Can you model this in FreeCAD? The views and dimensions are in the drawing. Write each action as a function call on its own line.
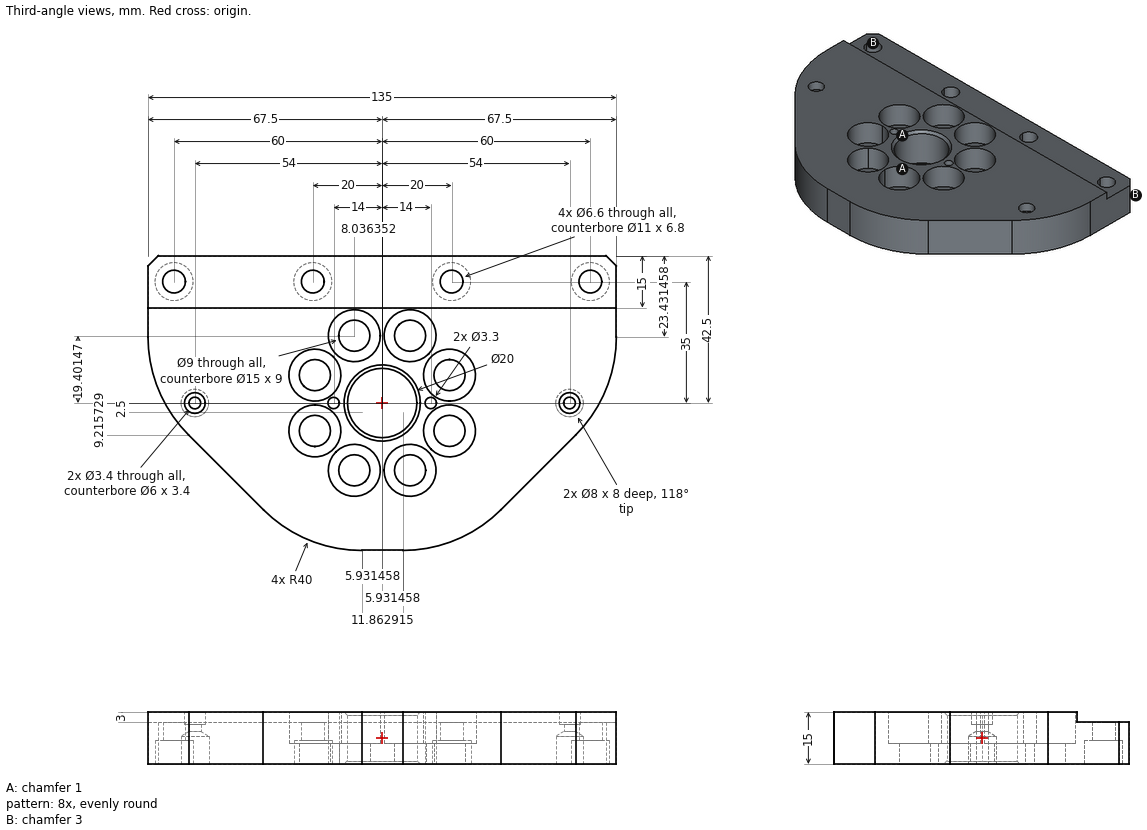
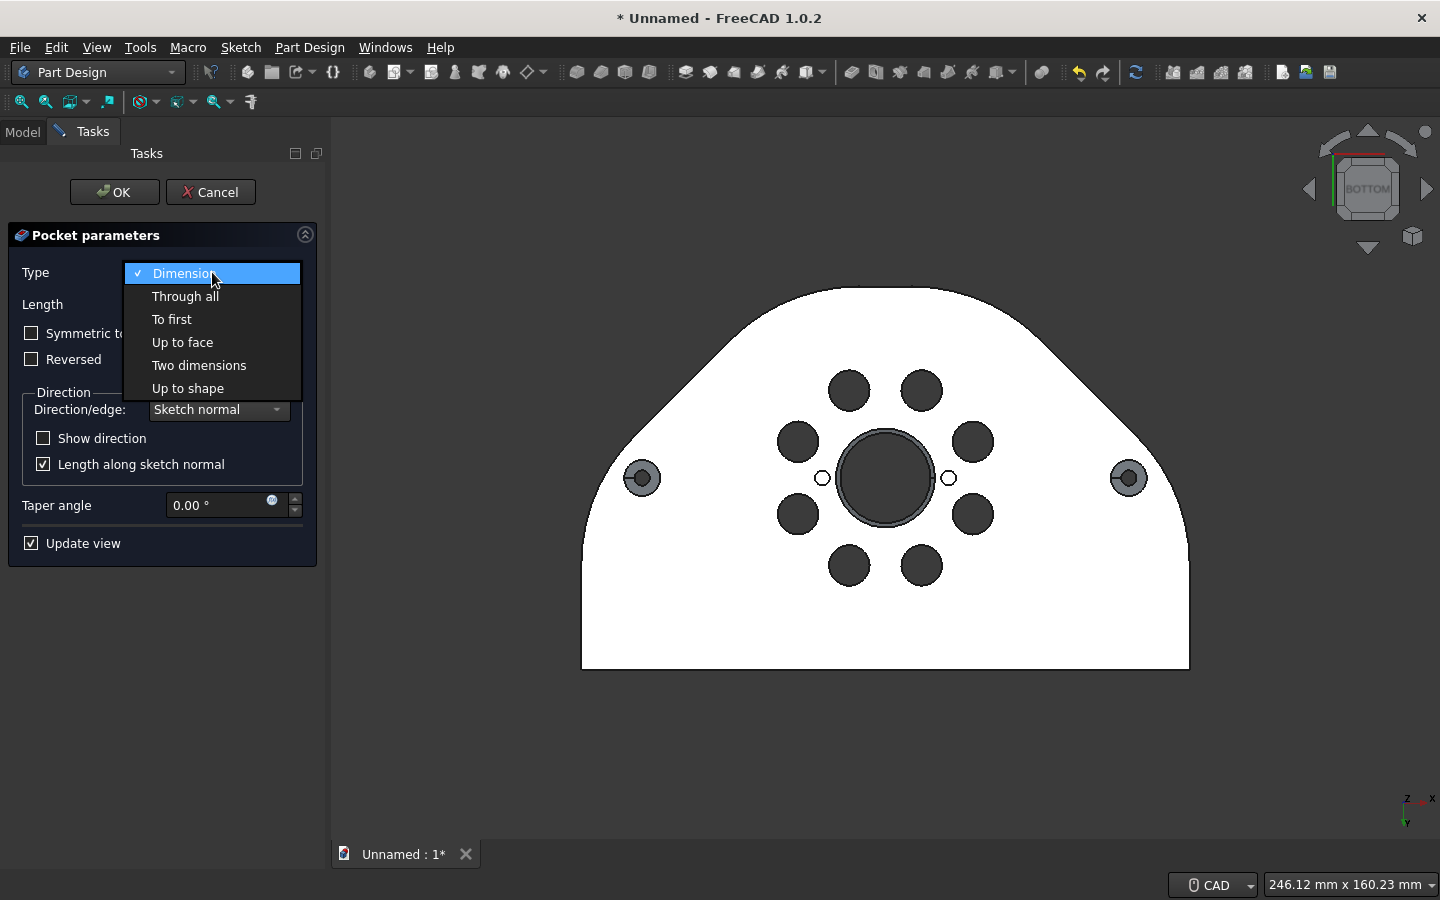
click(212, 296)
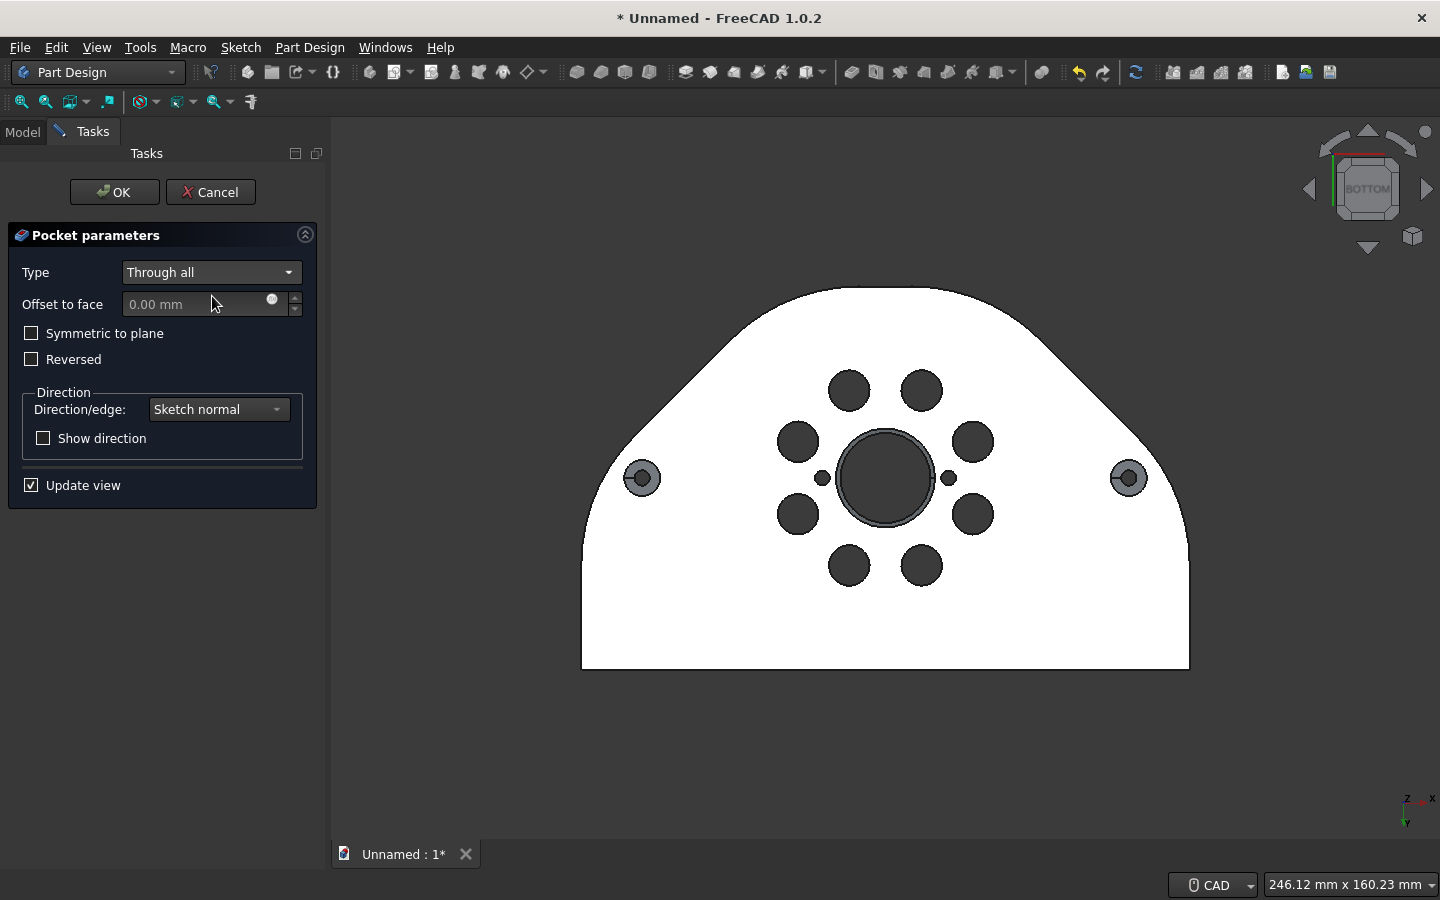
click(115, 192)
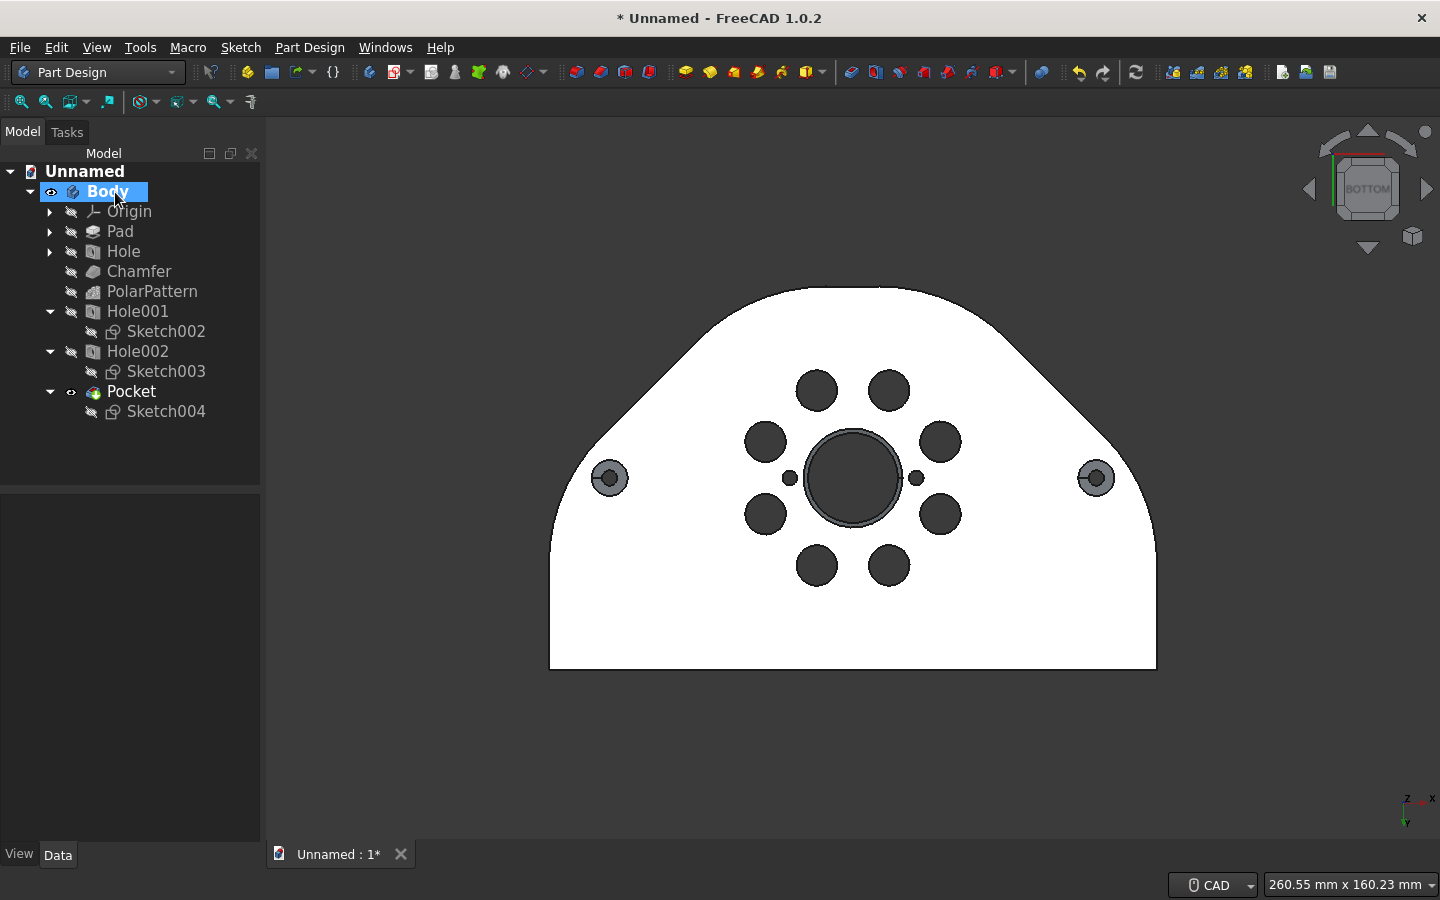
key(0)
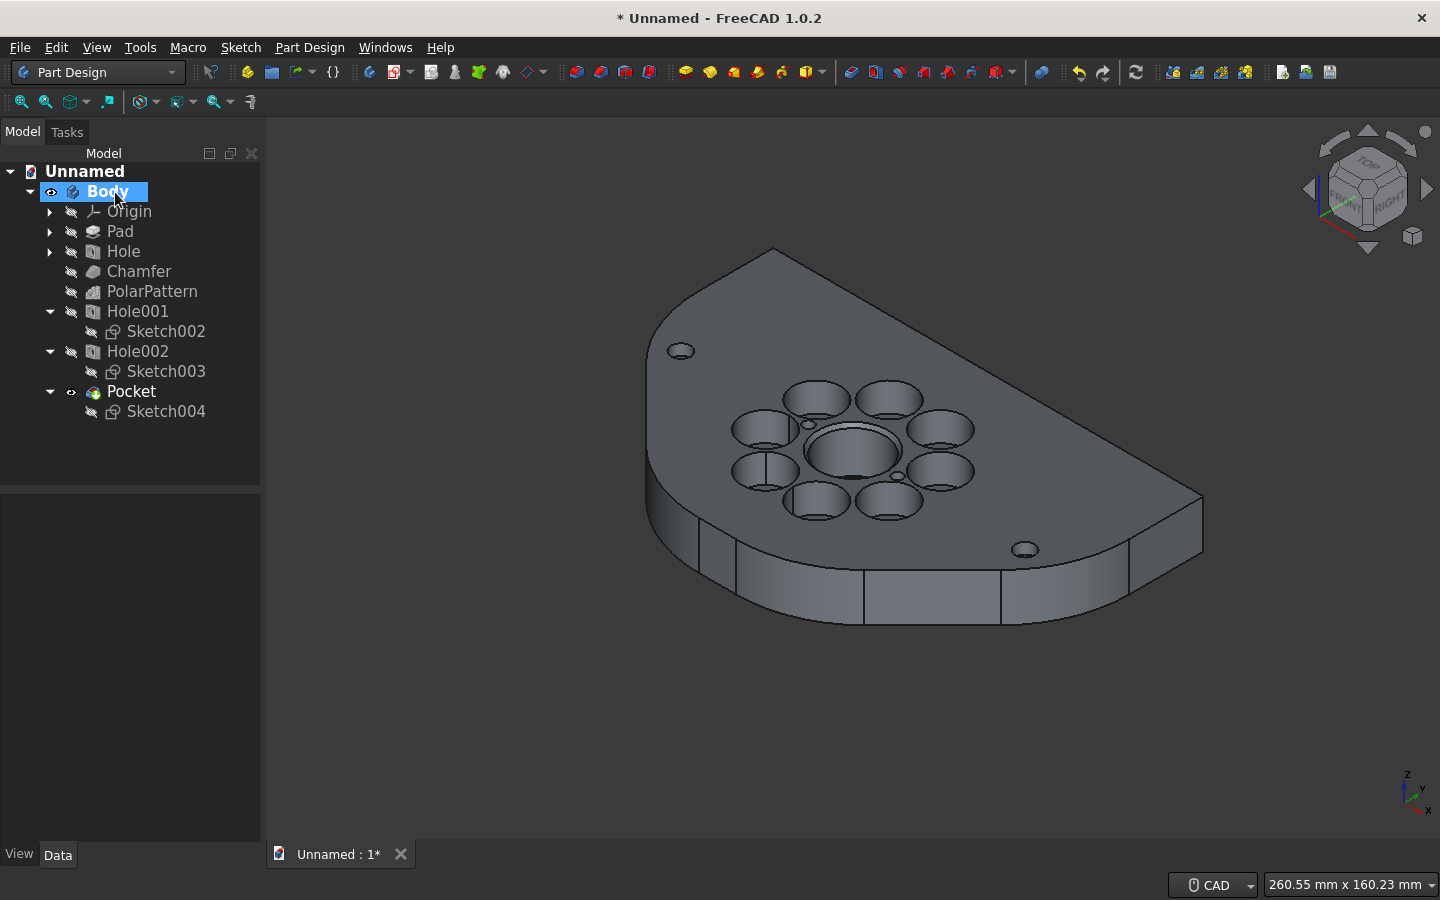
click(1053, 476)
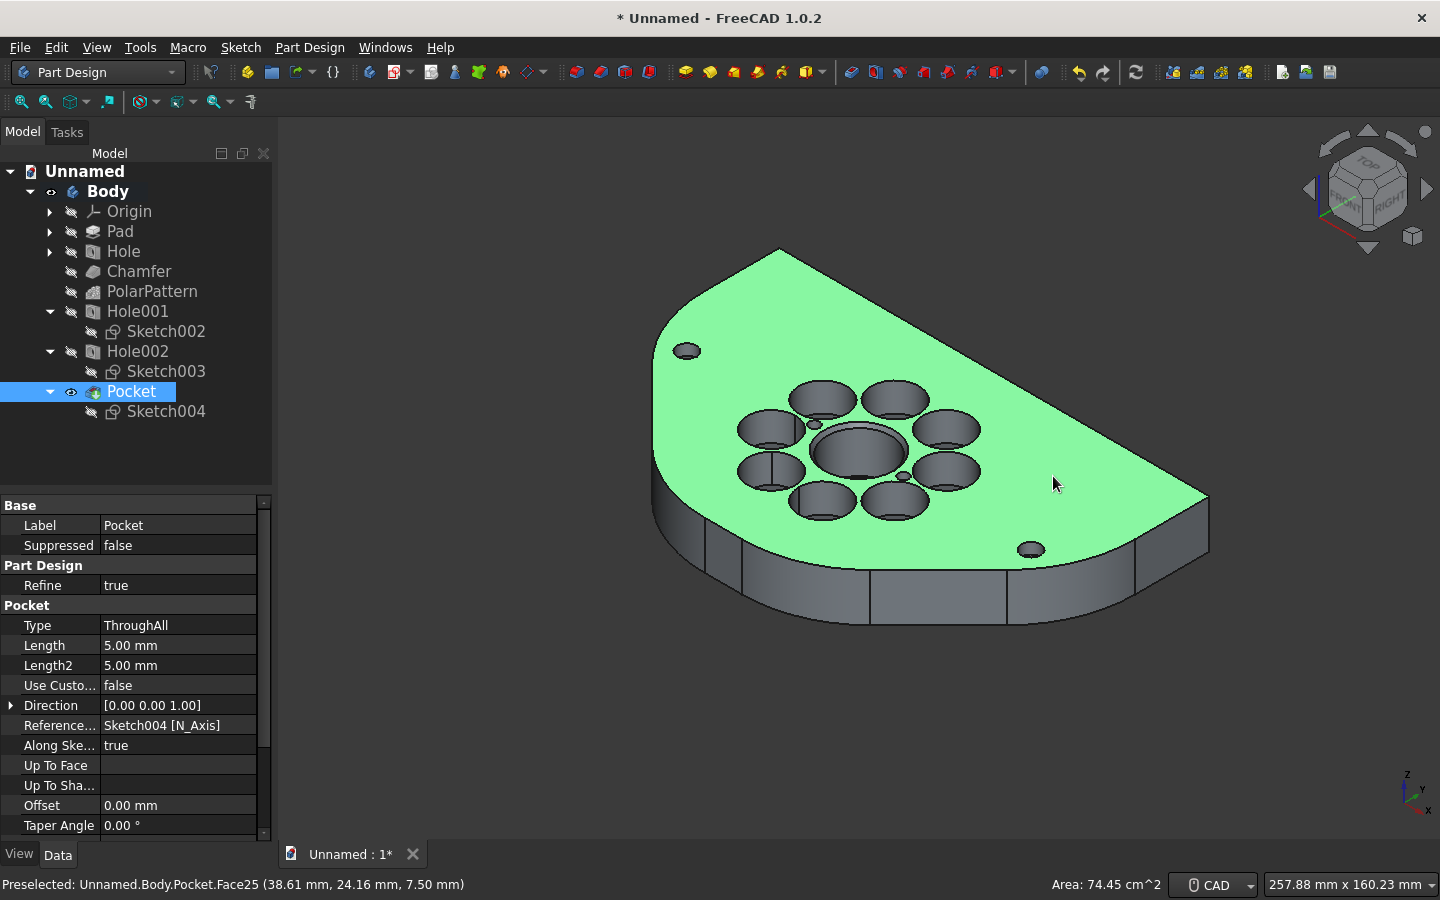
click(394, 72)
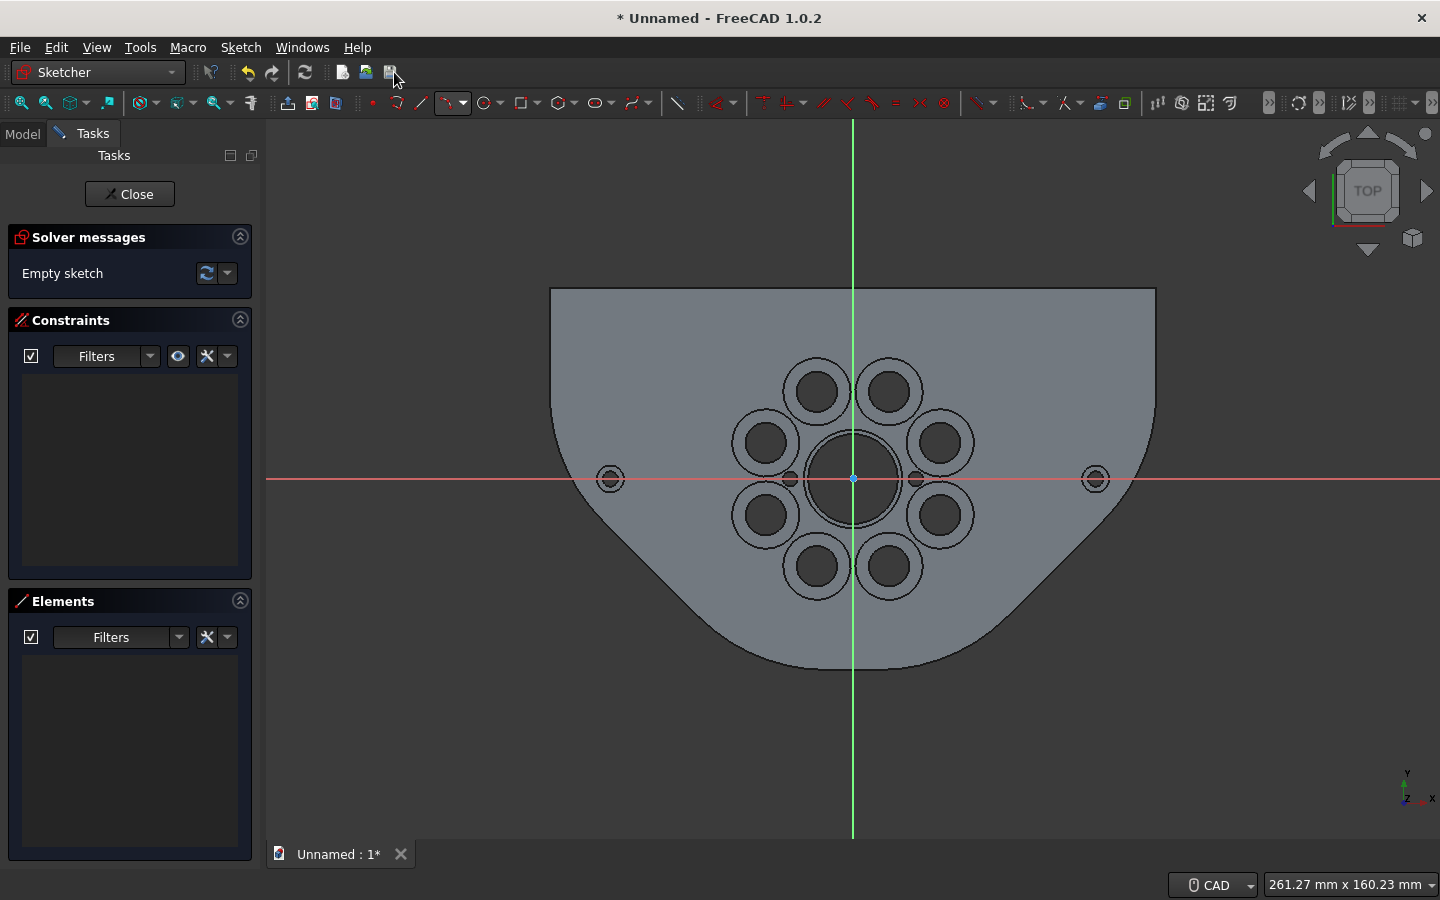
click(522, 104)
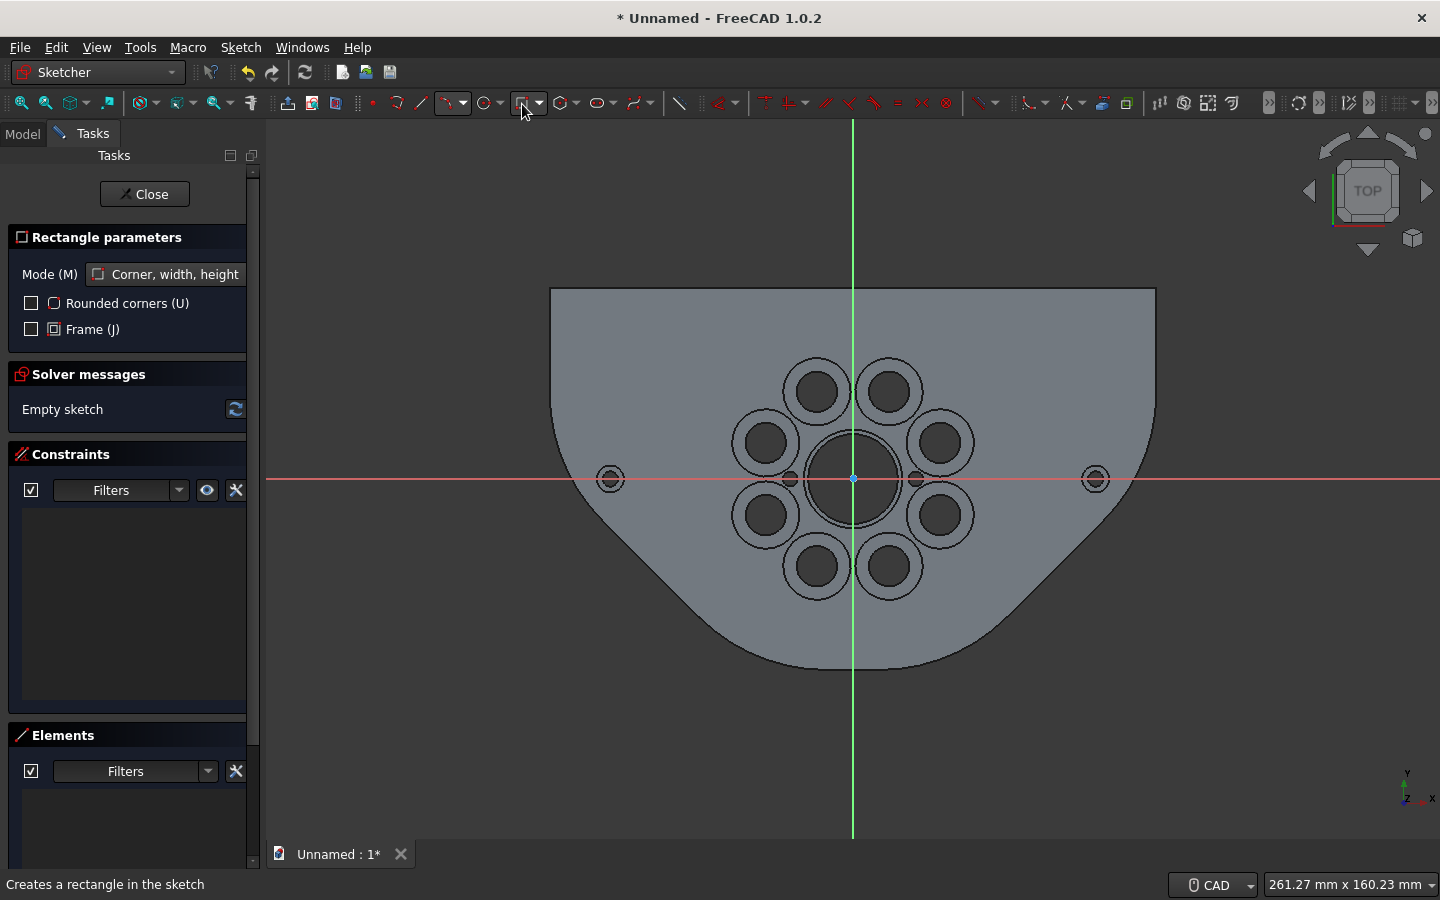
click(550, 288)
move(1156, 355)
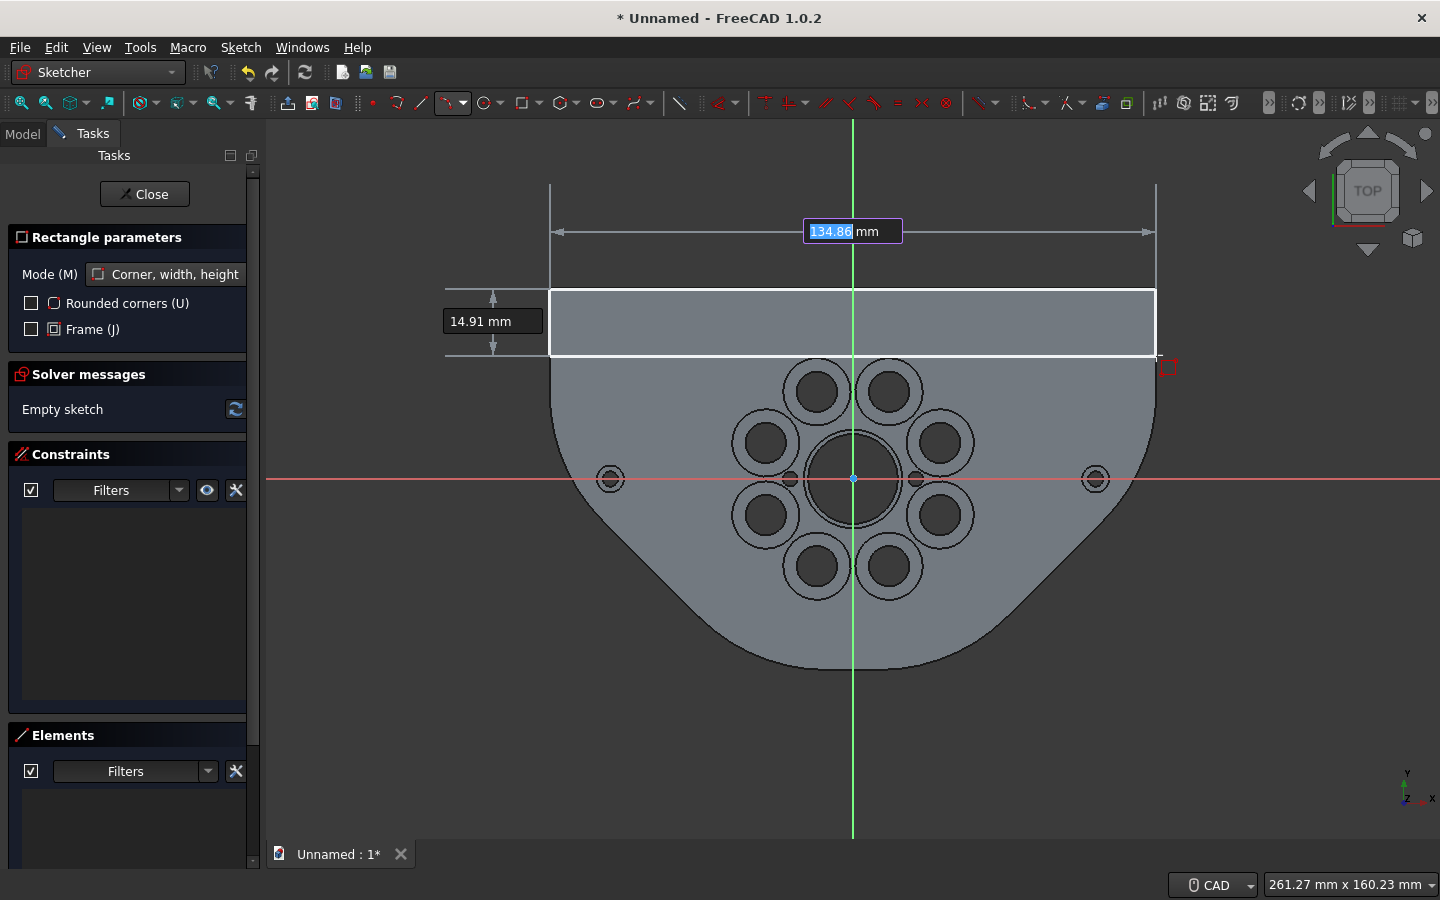
text(135)
key(Tab)
text(15)
key(Return)
key(Escape)